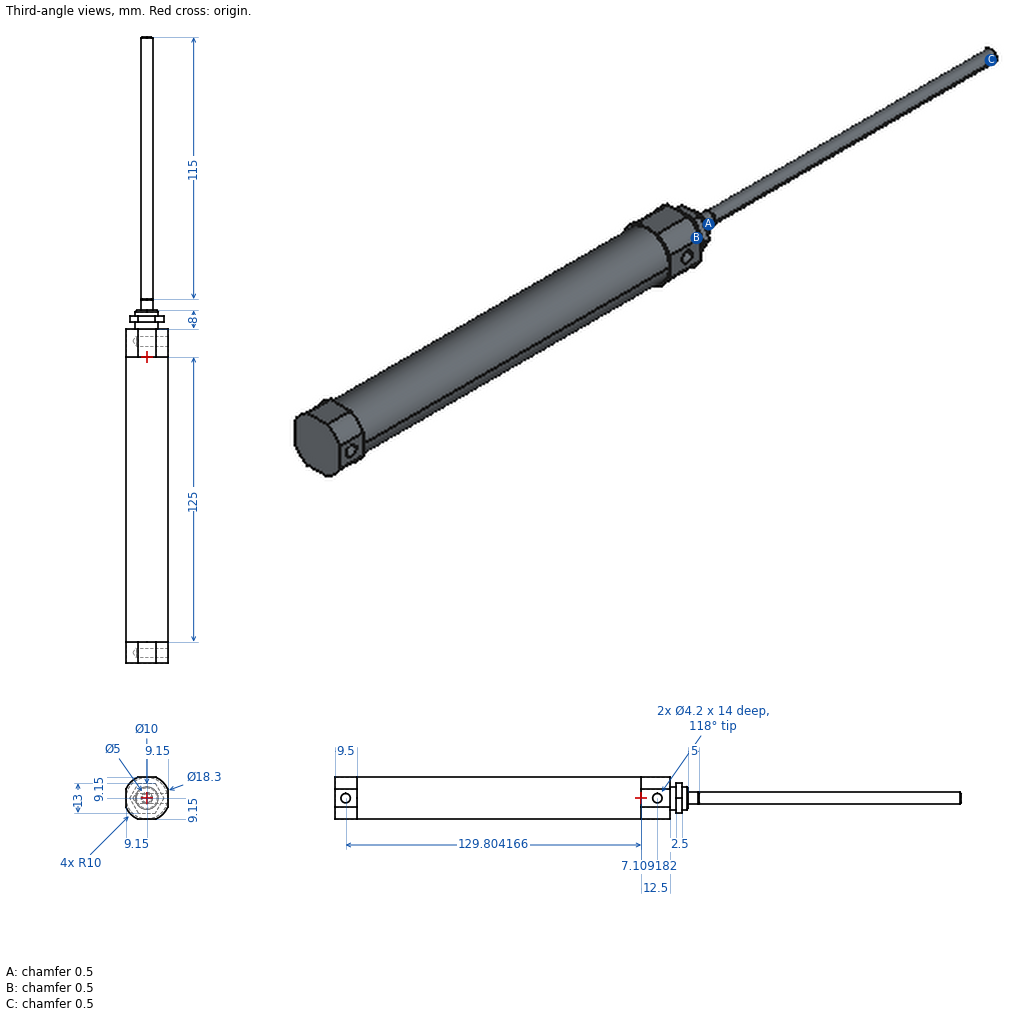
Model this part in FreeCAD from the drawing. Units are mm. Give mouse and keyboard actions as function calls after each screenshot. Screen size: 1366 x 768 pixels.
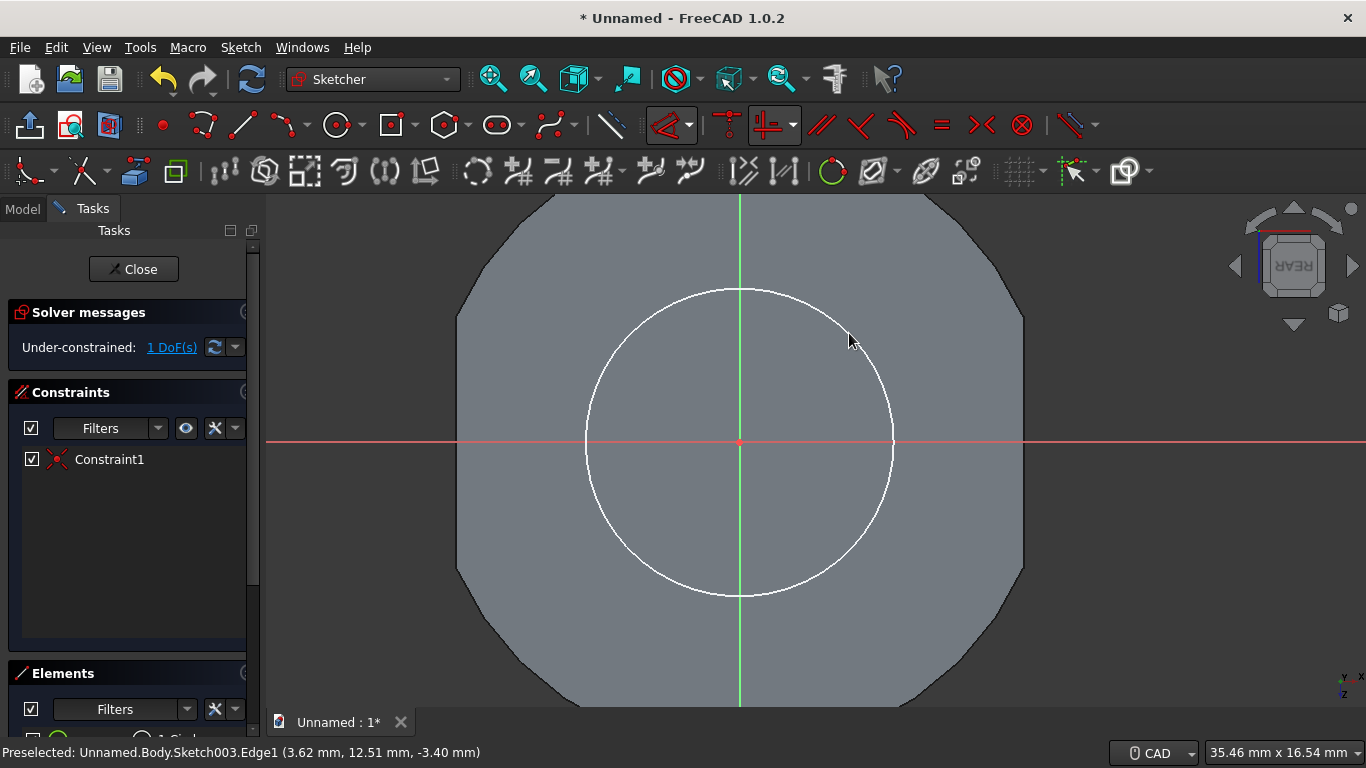
key(d)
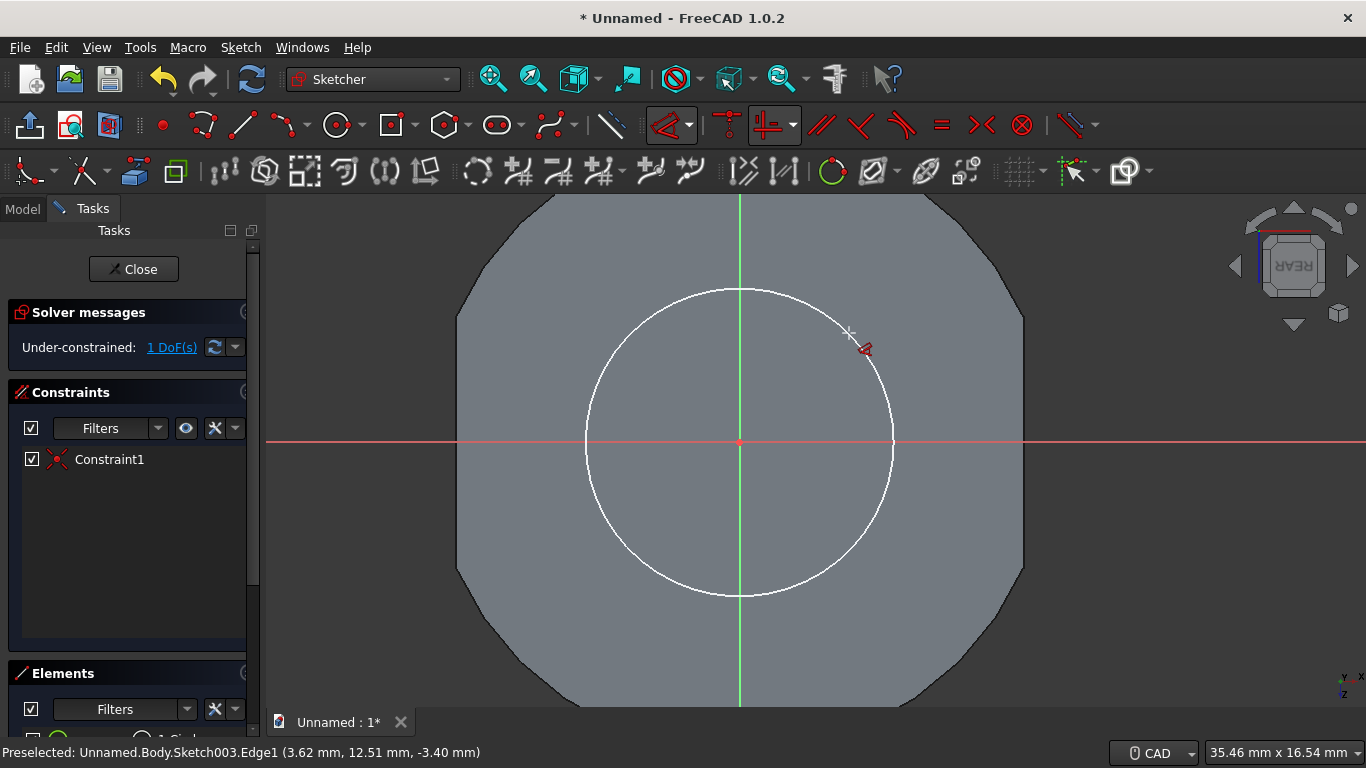
click(848, 333)
click(871, 310)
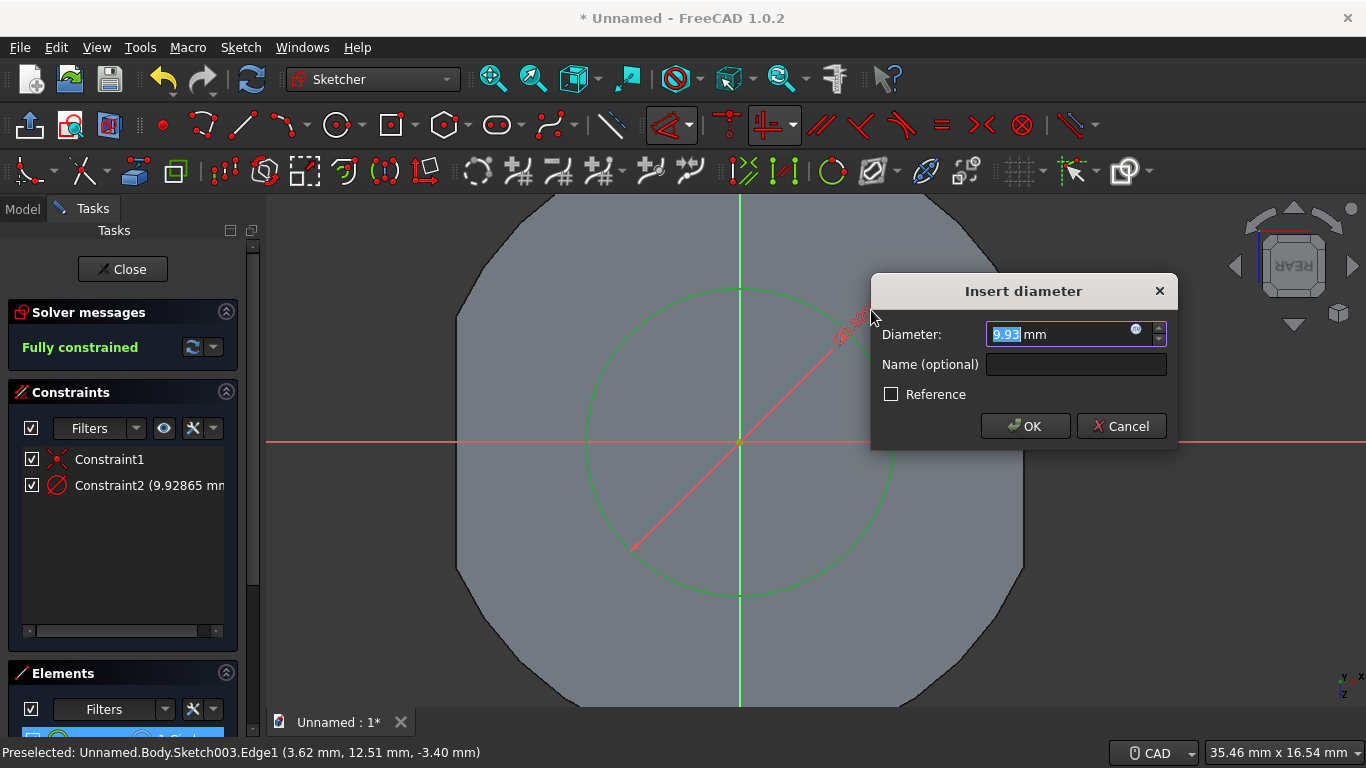
text(10)
key(Return)
key(Escape)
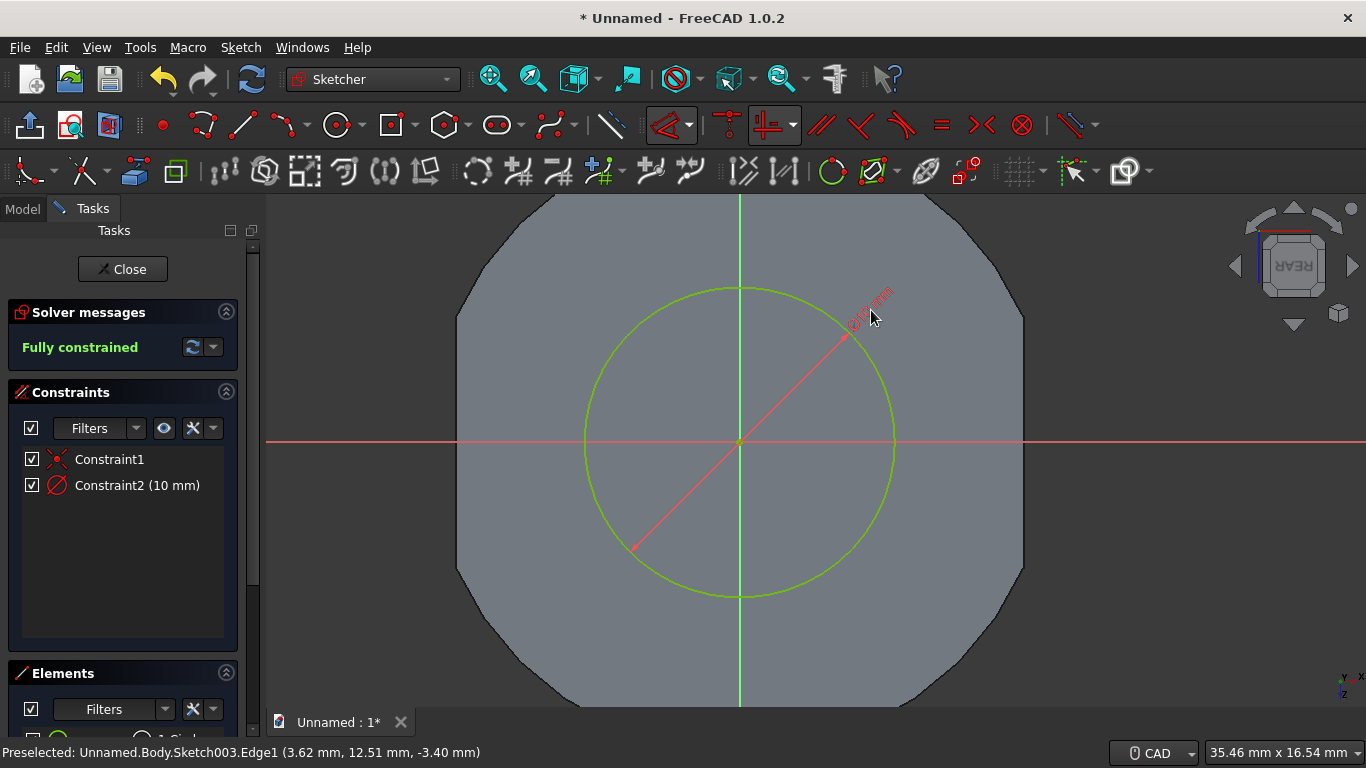
click(123, 269)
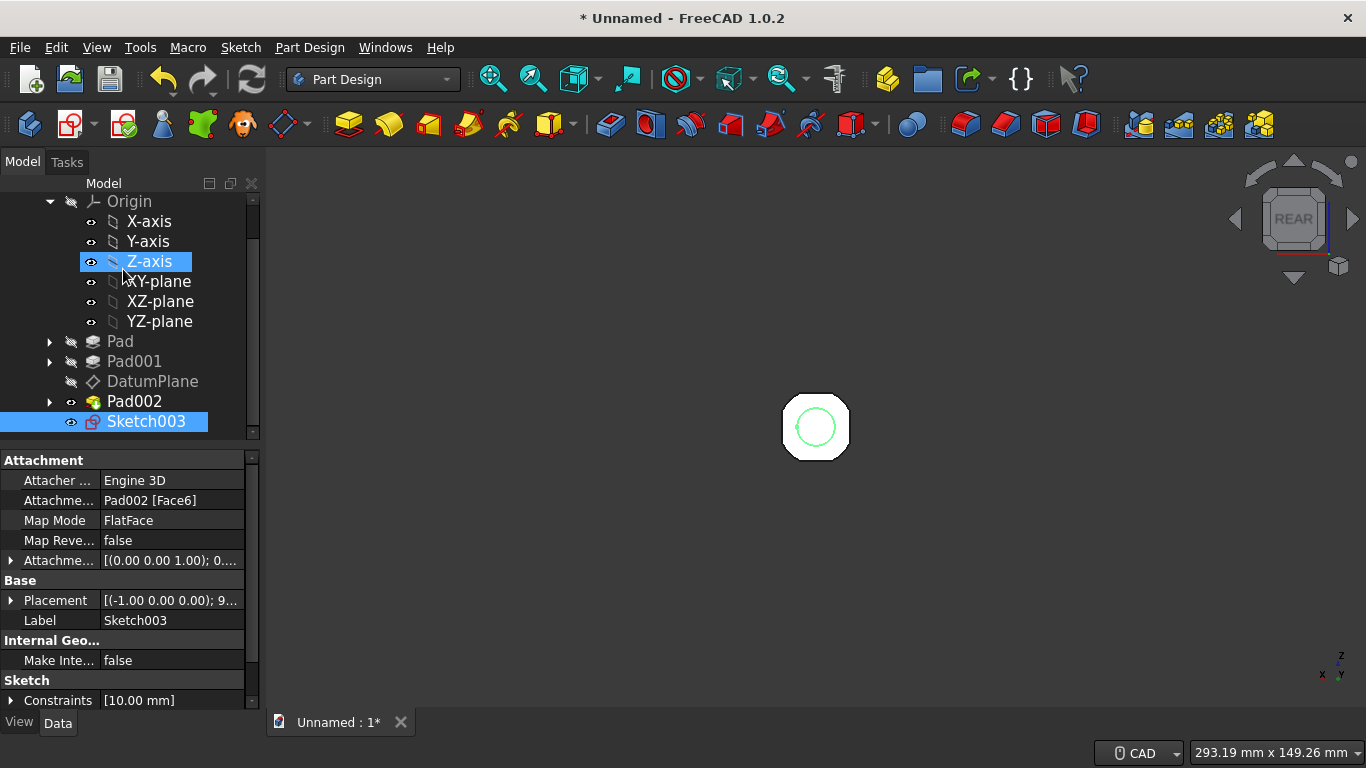
click(350, 124)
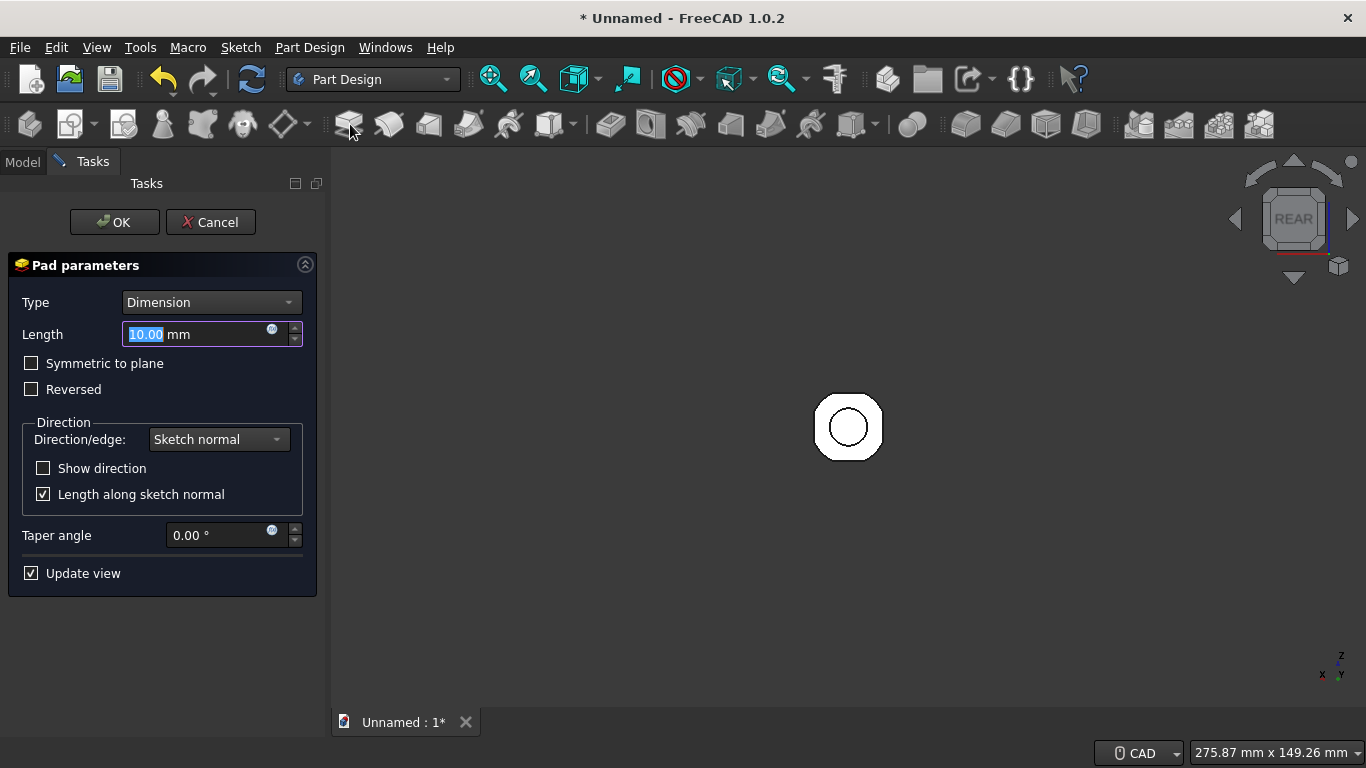
text(8)
key(Tab)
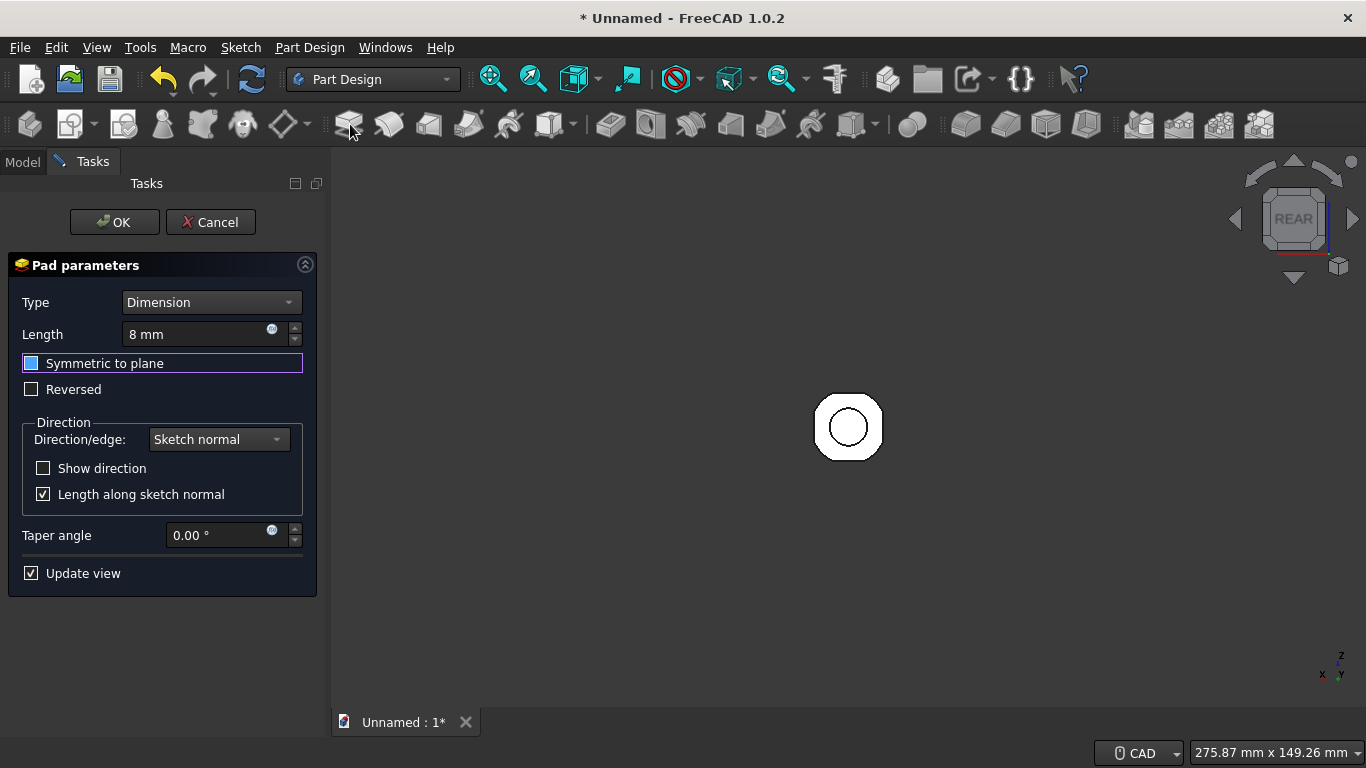
click(115, 222)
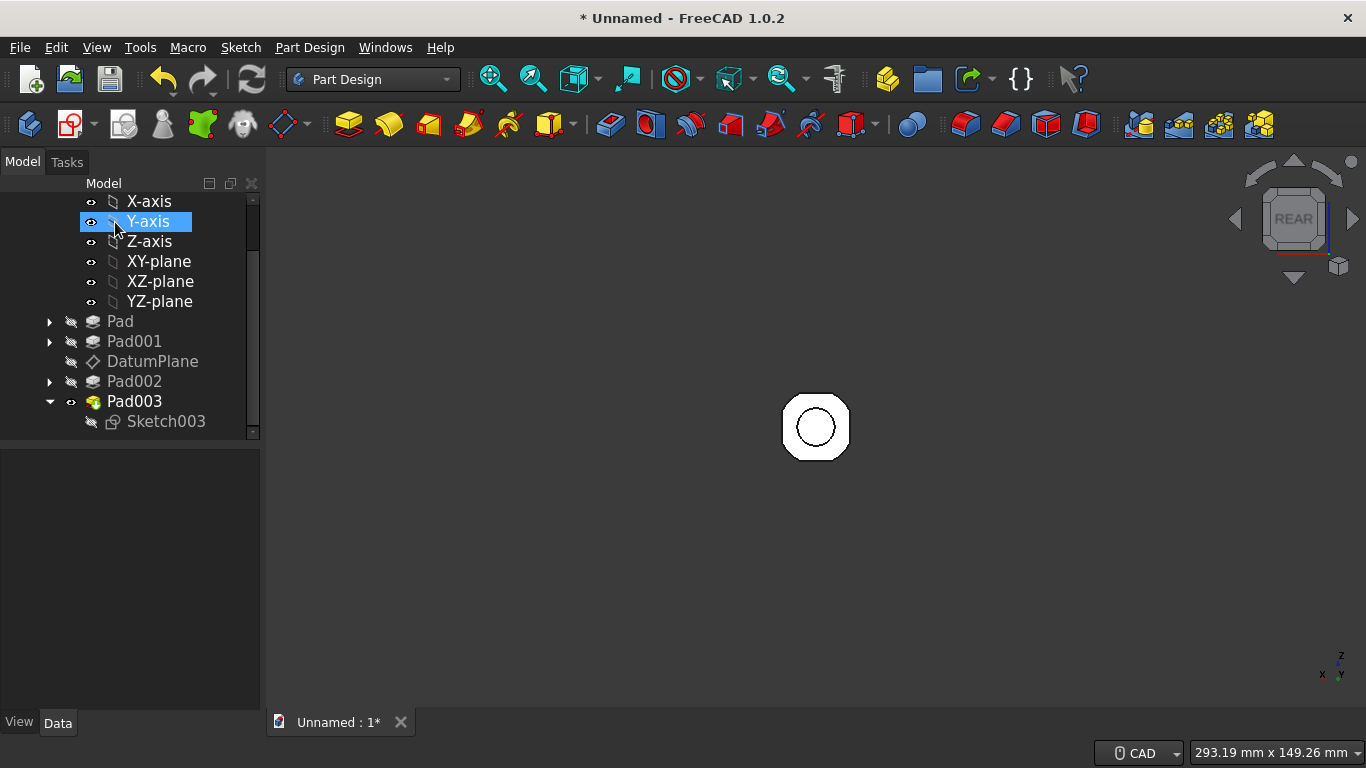
key(v)
key(f)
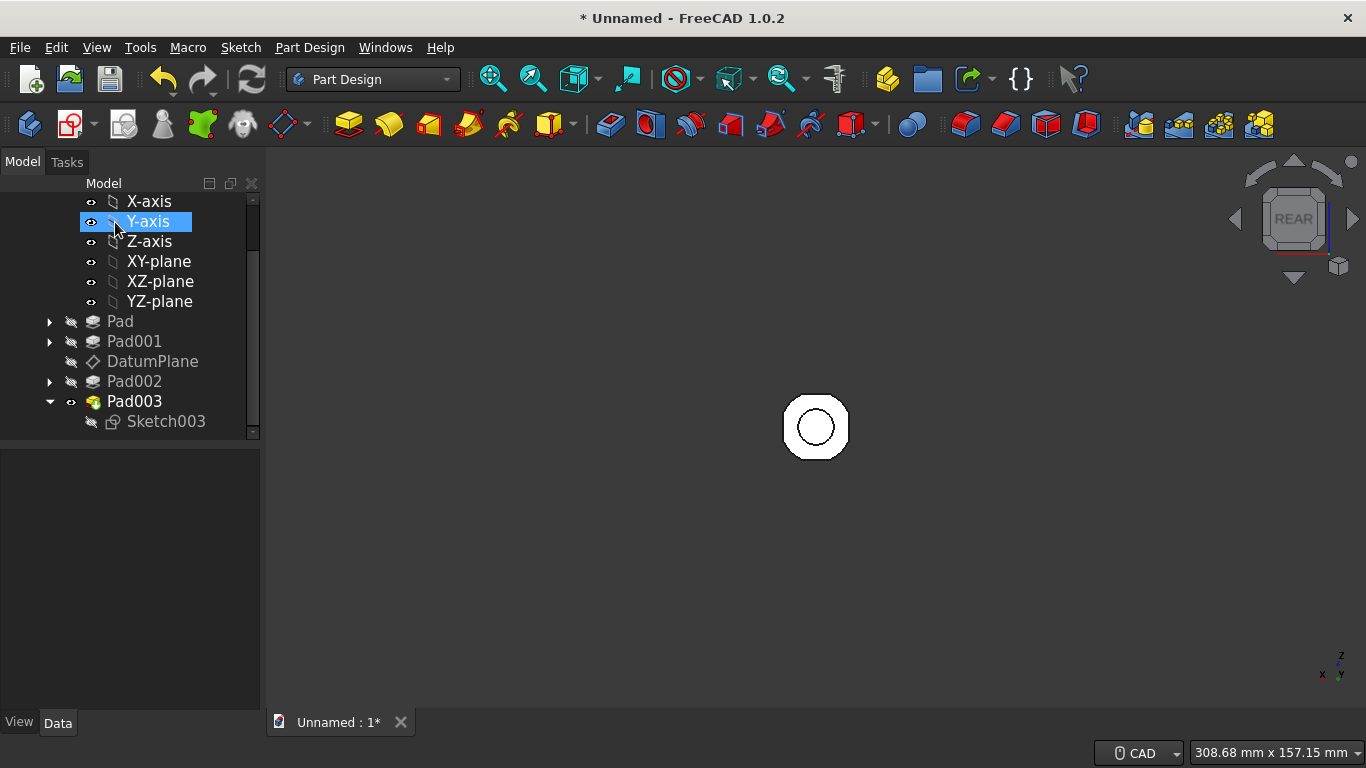
click(816, 426)